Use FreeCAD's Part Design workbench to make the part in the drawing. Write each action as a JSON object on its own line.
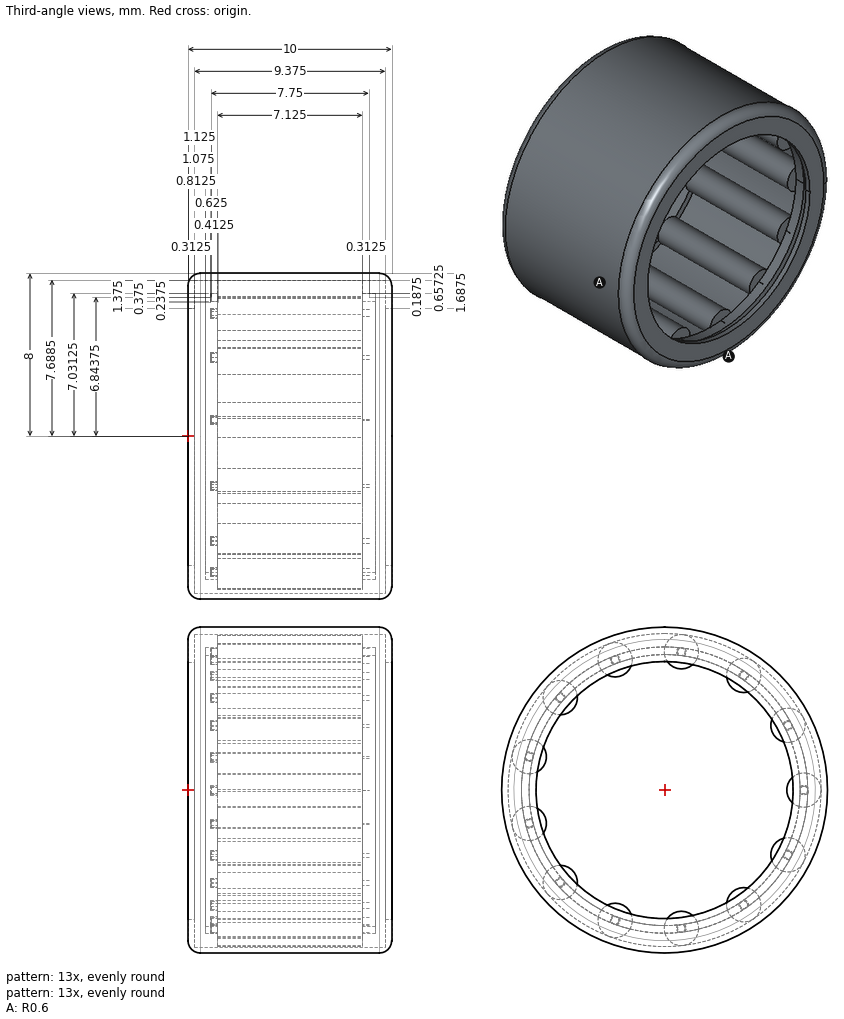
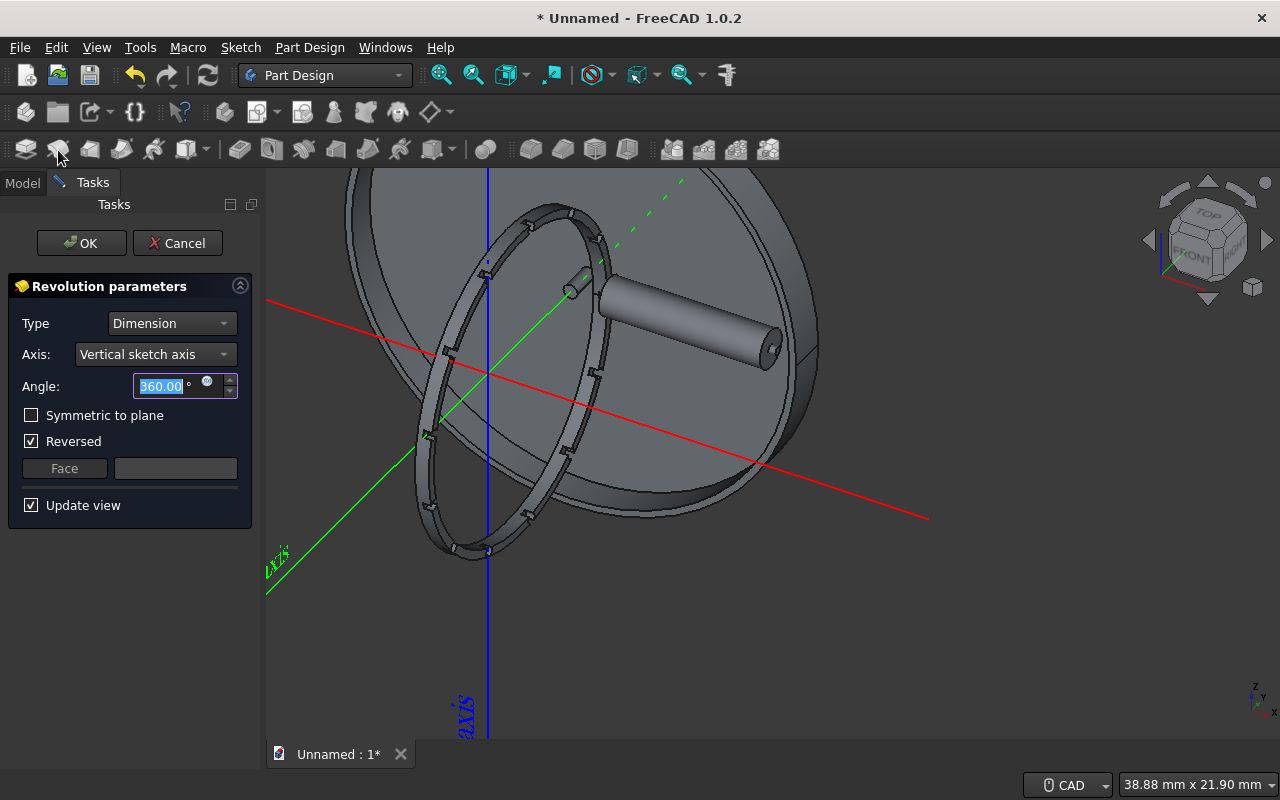
{"action": "left_click", "coordinate": [156, 354]}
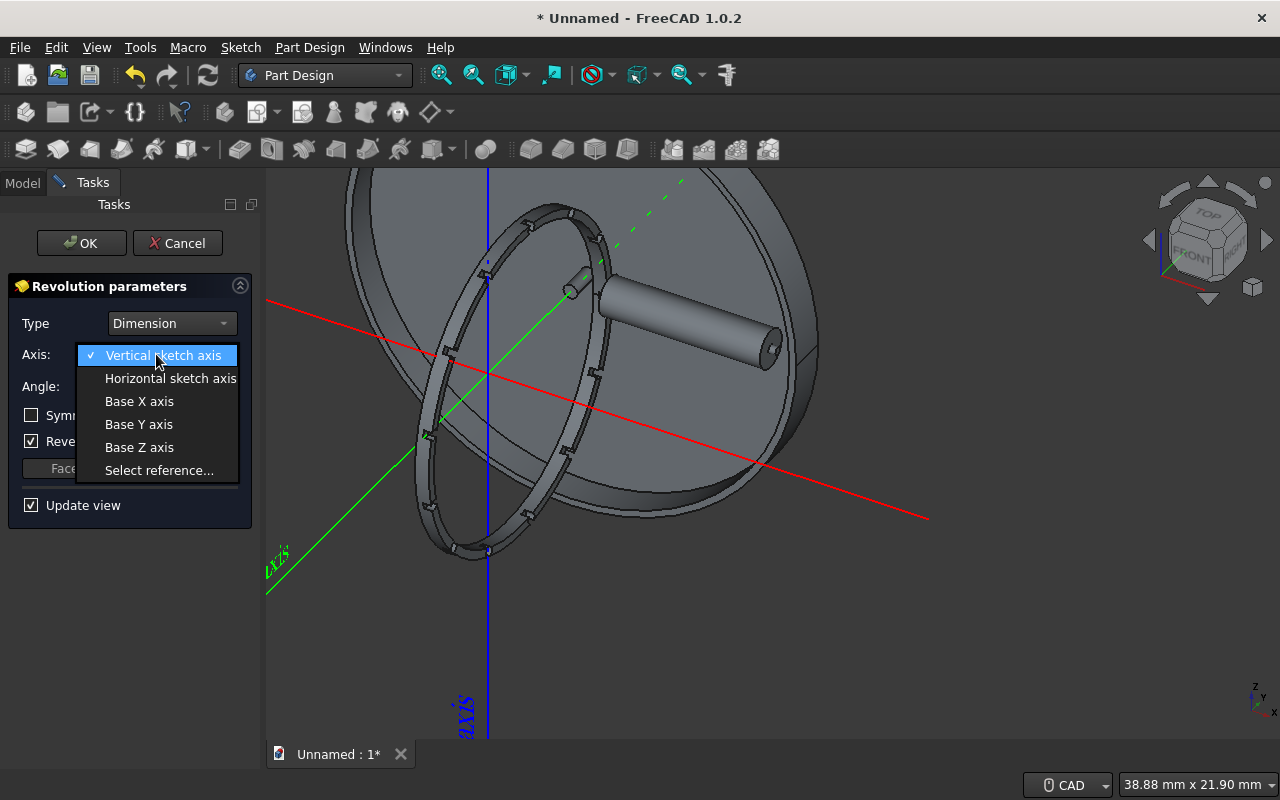
{"action": "left_click", "coordinate": [156, 378]}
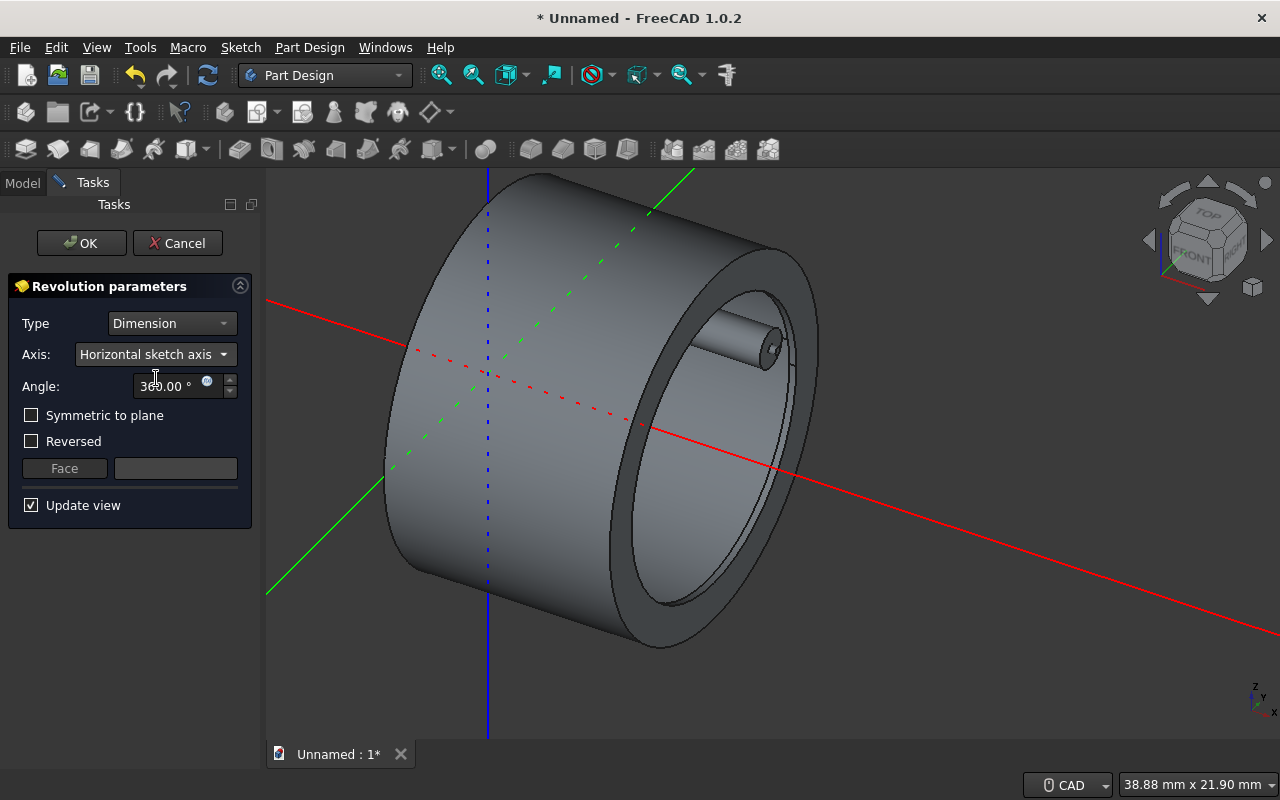
{"action": "left_click", "coordinate": [82, 243]}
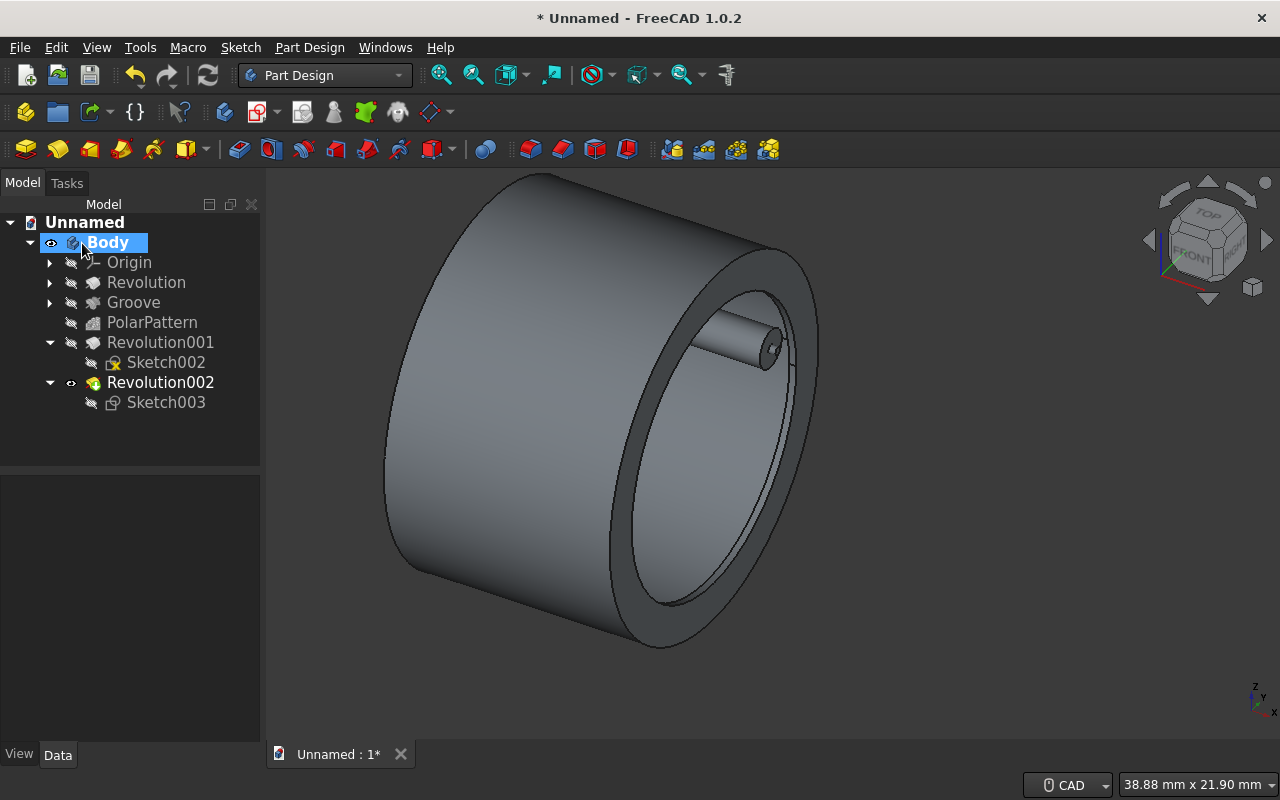
{"action": "left_click", "coordinate": [442, 76]}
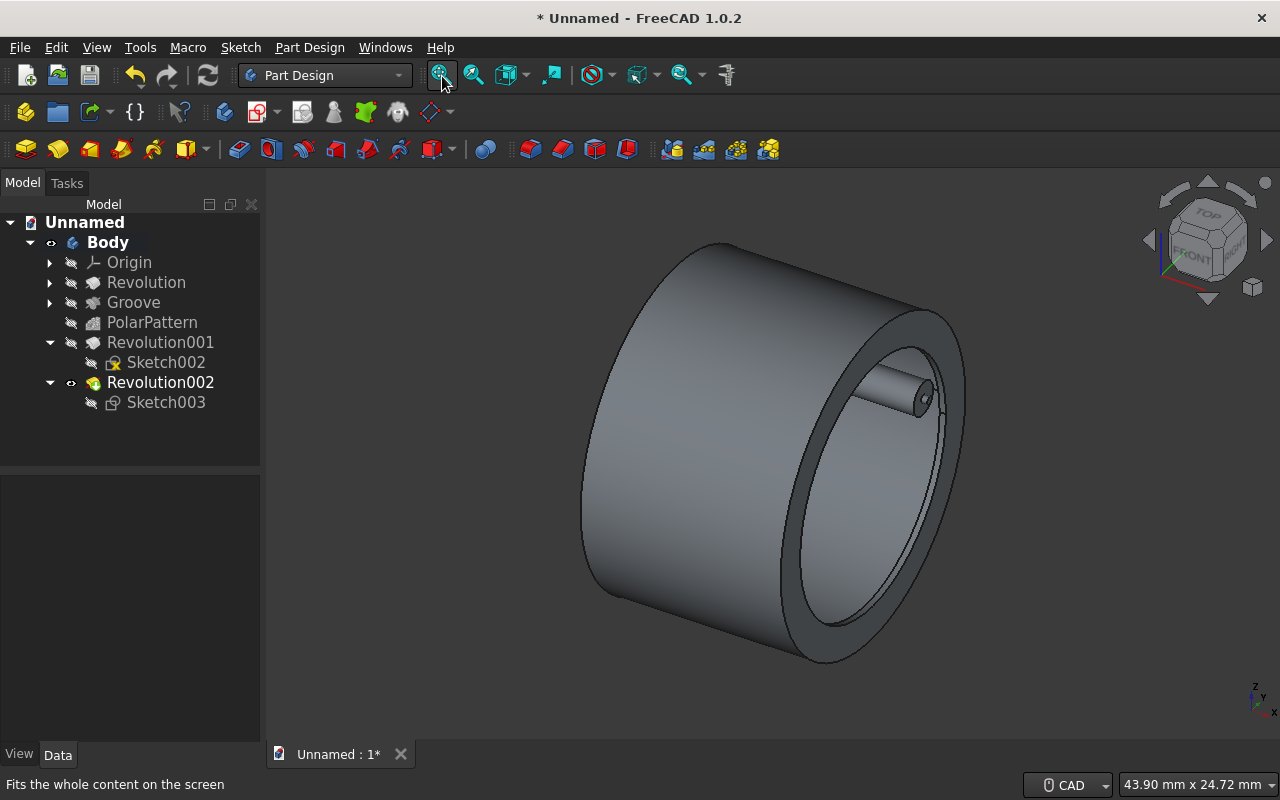
{"action": "left_click", "coordinate": [50, 263]}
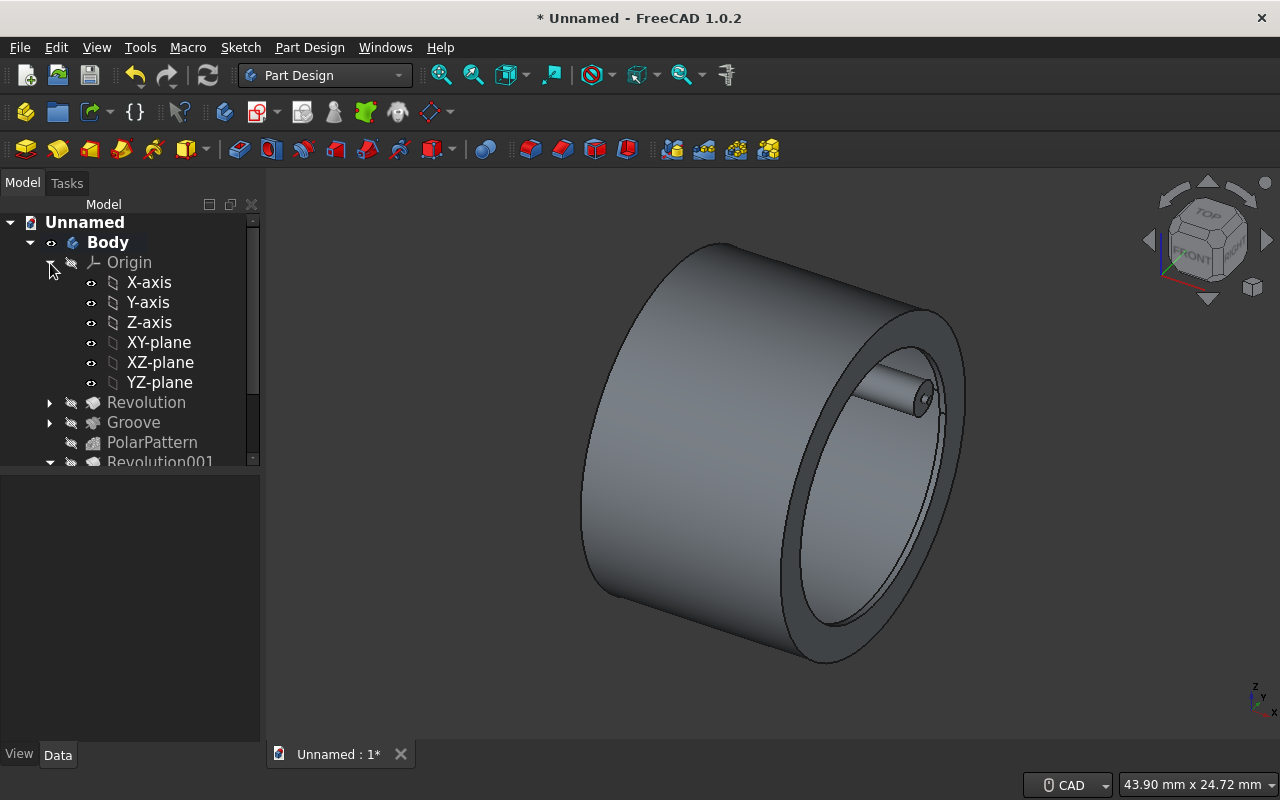
{"action": "left_click", "coordinate": [136, 383]}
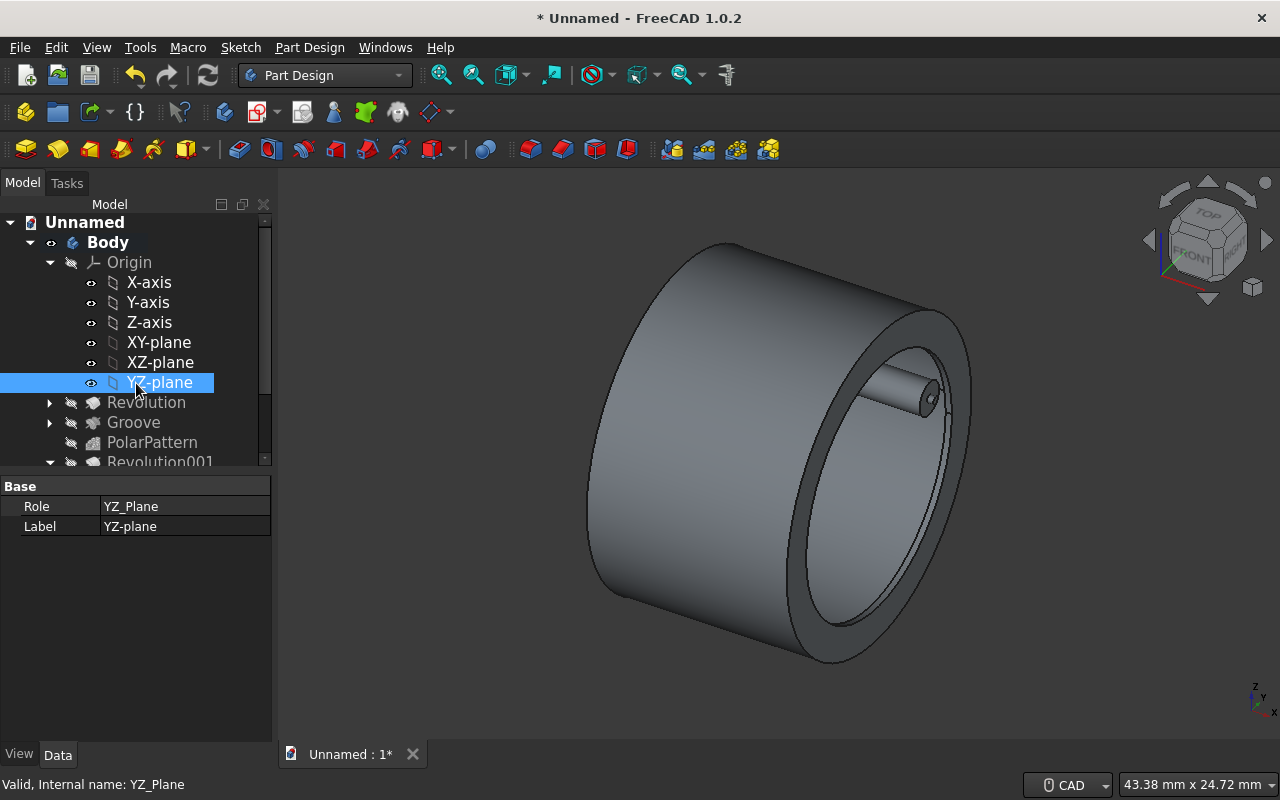
{"action": "left_click", "coordinate": [430, 112]}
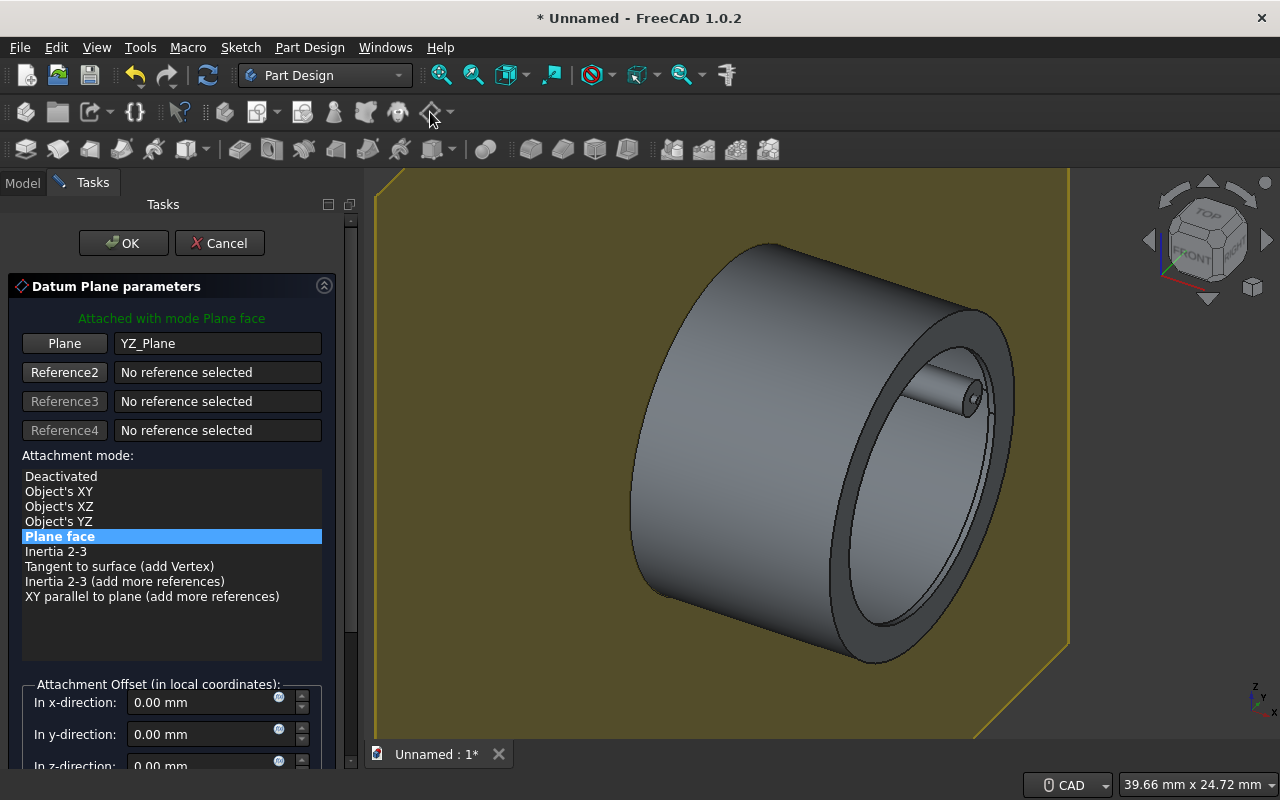
{"action": "scroll", "coordinate": [351, 491], "scroll_direction": "down", "scroll_amount": 2}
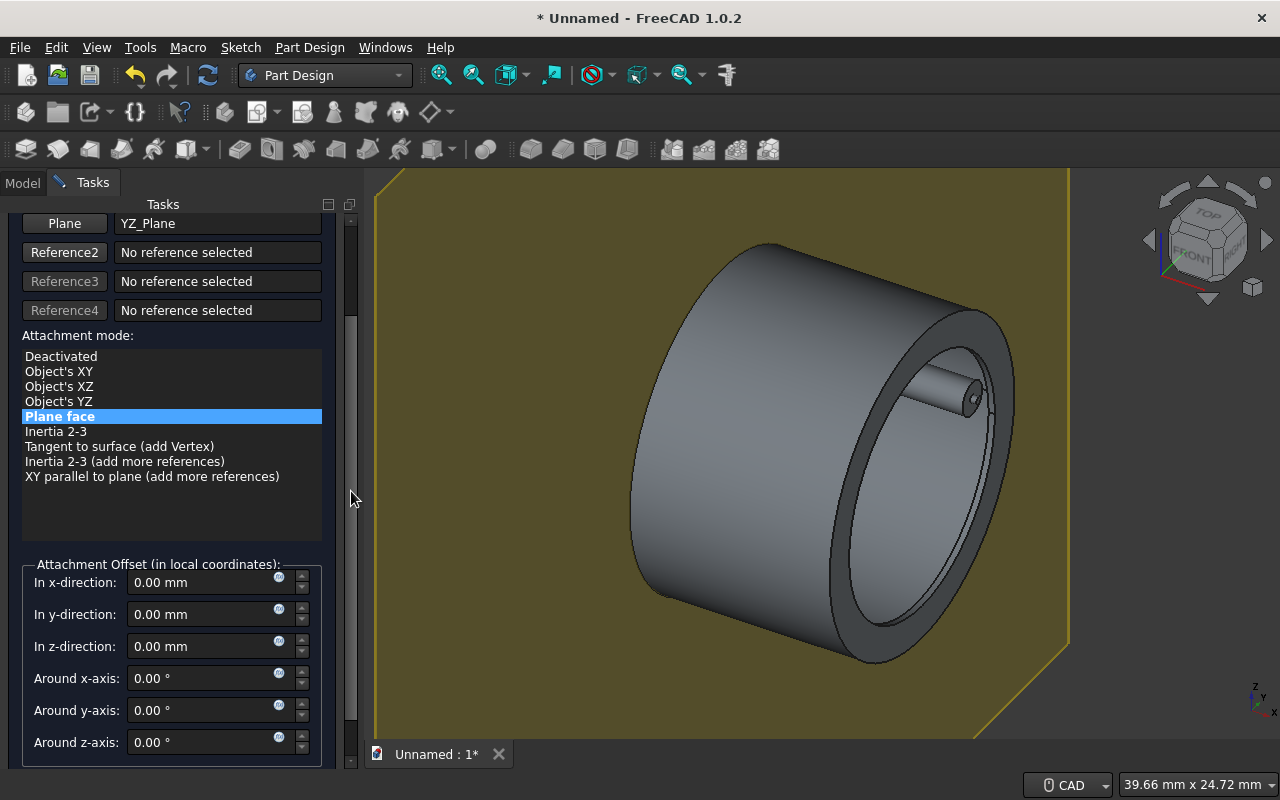
{"action": "triple_click", "coordinate": [210, 646]}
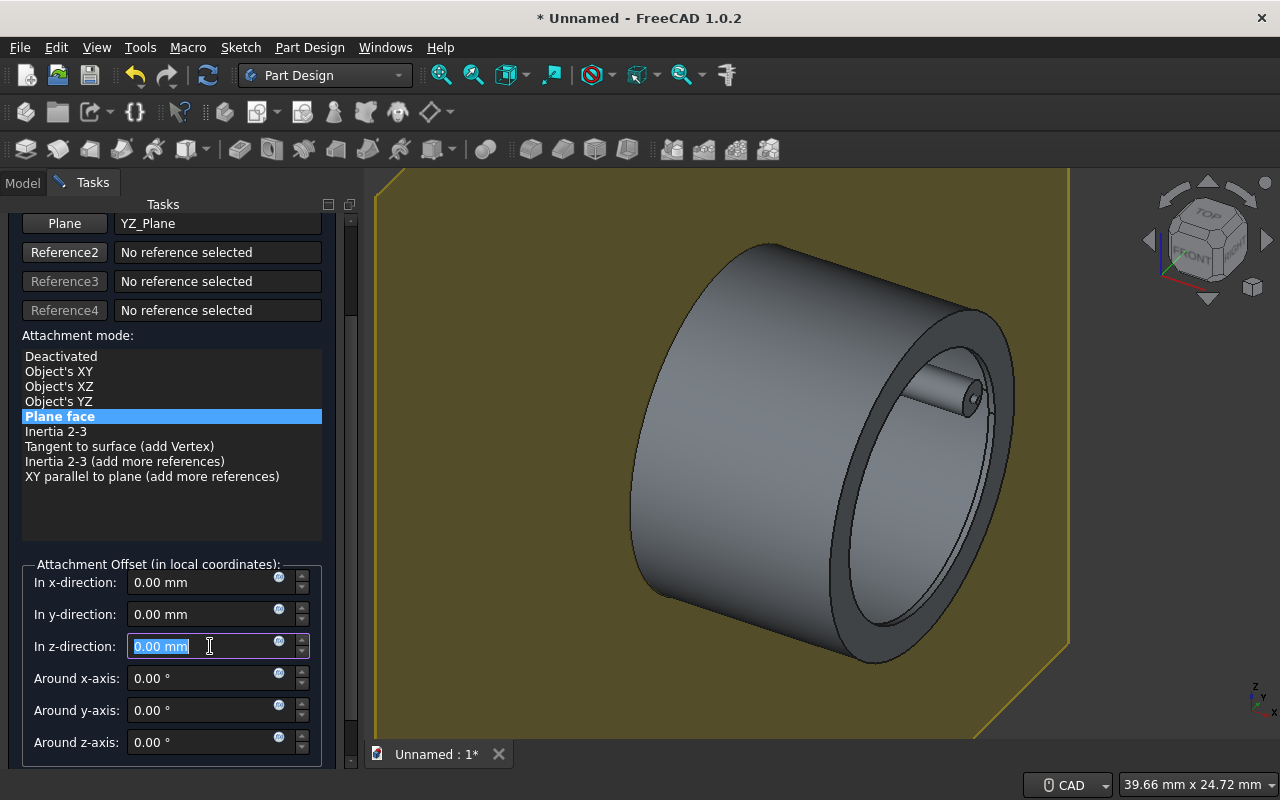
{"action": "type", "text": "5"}
{"action": "key", "text": "Tab"}